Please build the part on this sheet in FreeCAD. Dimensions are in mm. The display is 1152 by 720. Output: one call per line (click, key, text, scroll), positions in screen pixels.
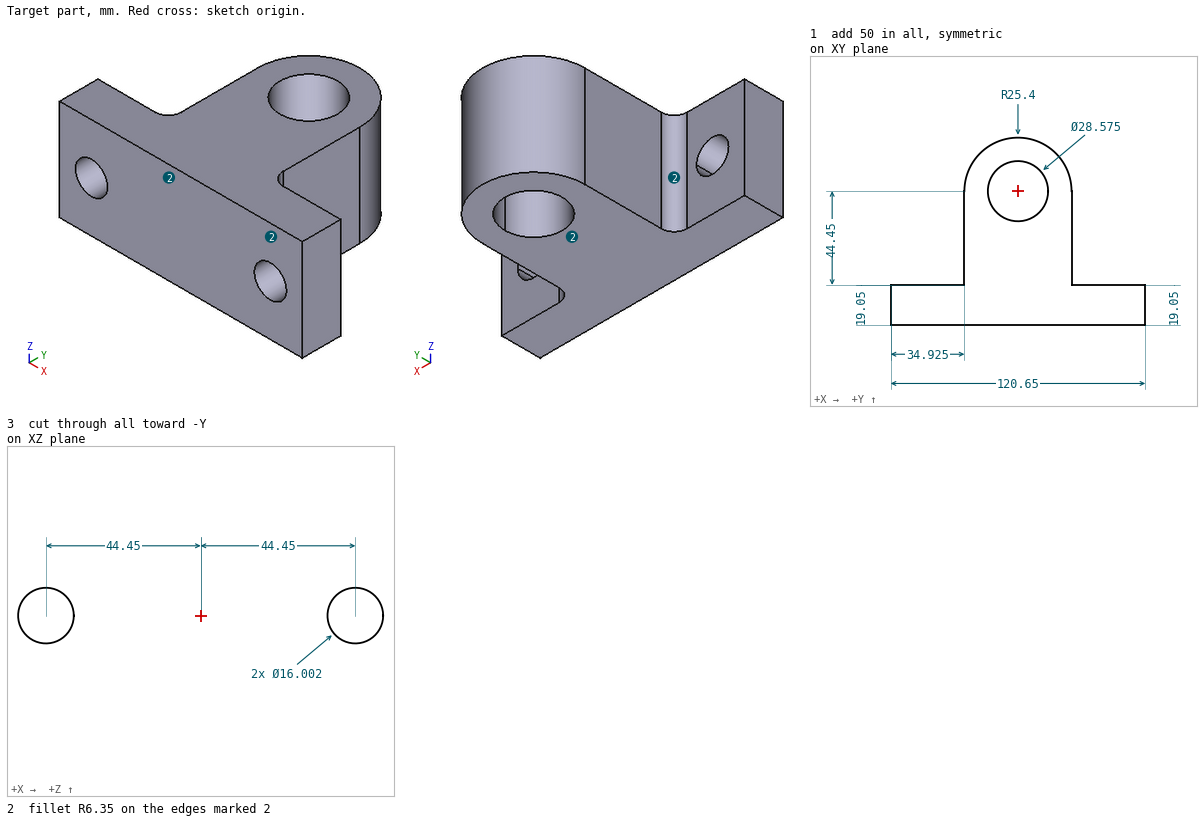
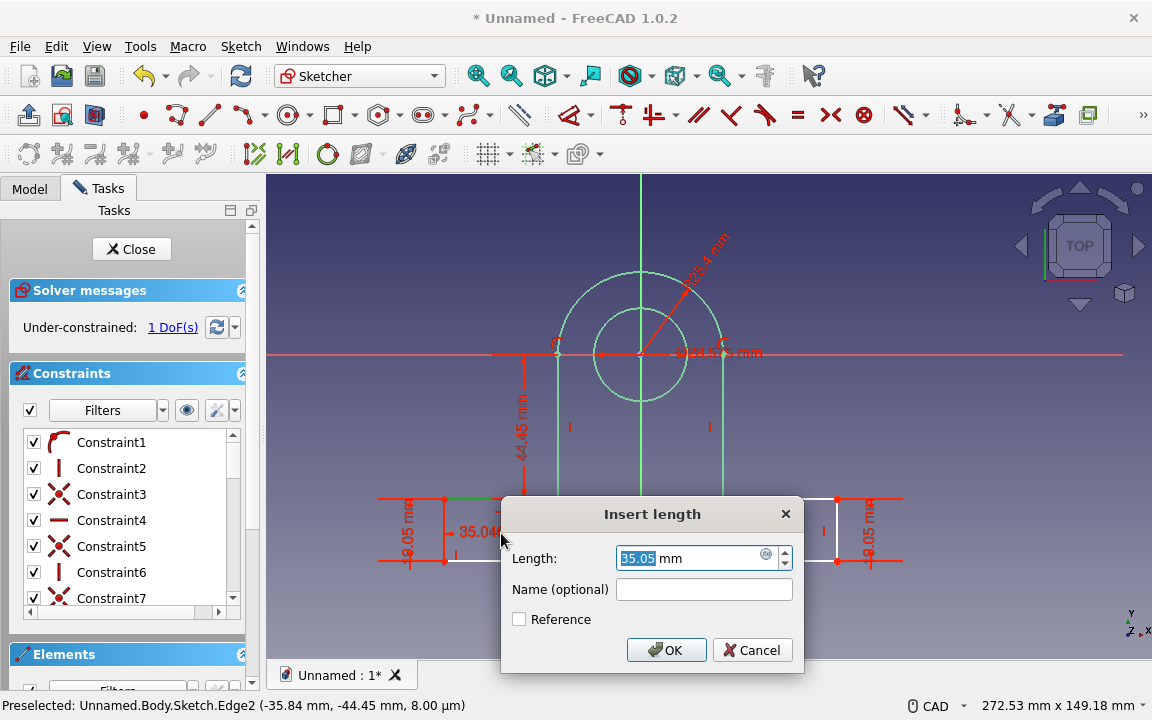
text(34.925)
key(Return)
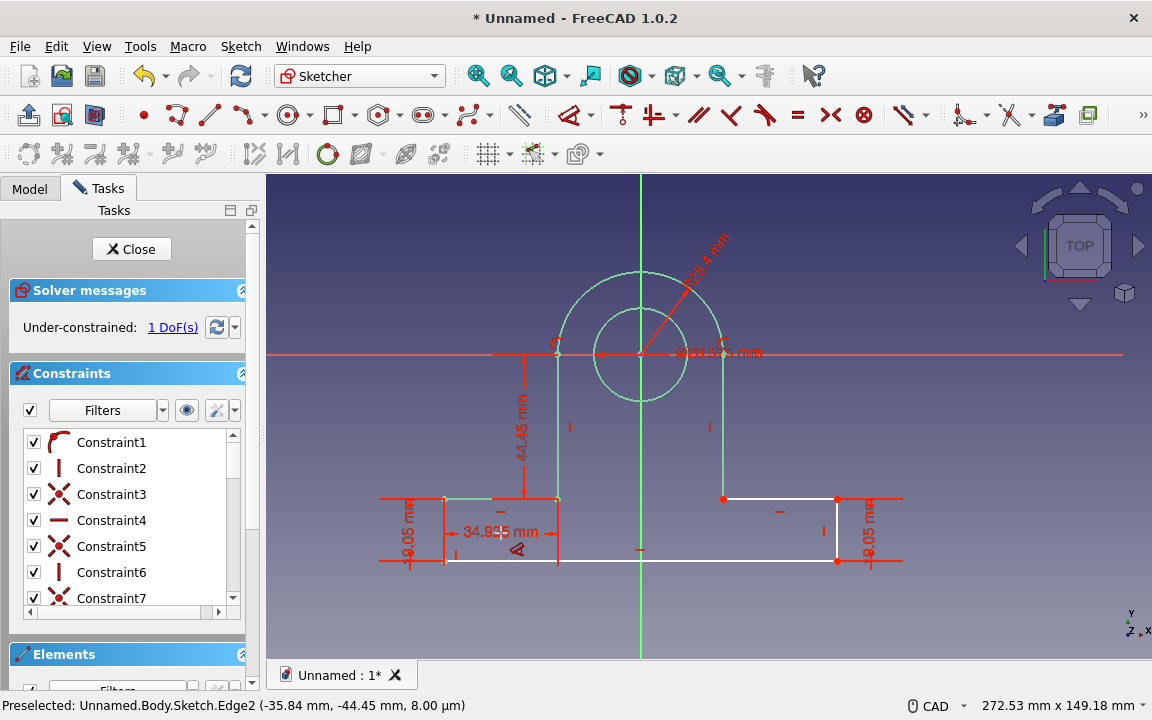
click(562, 561)
click(550, 595)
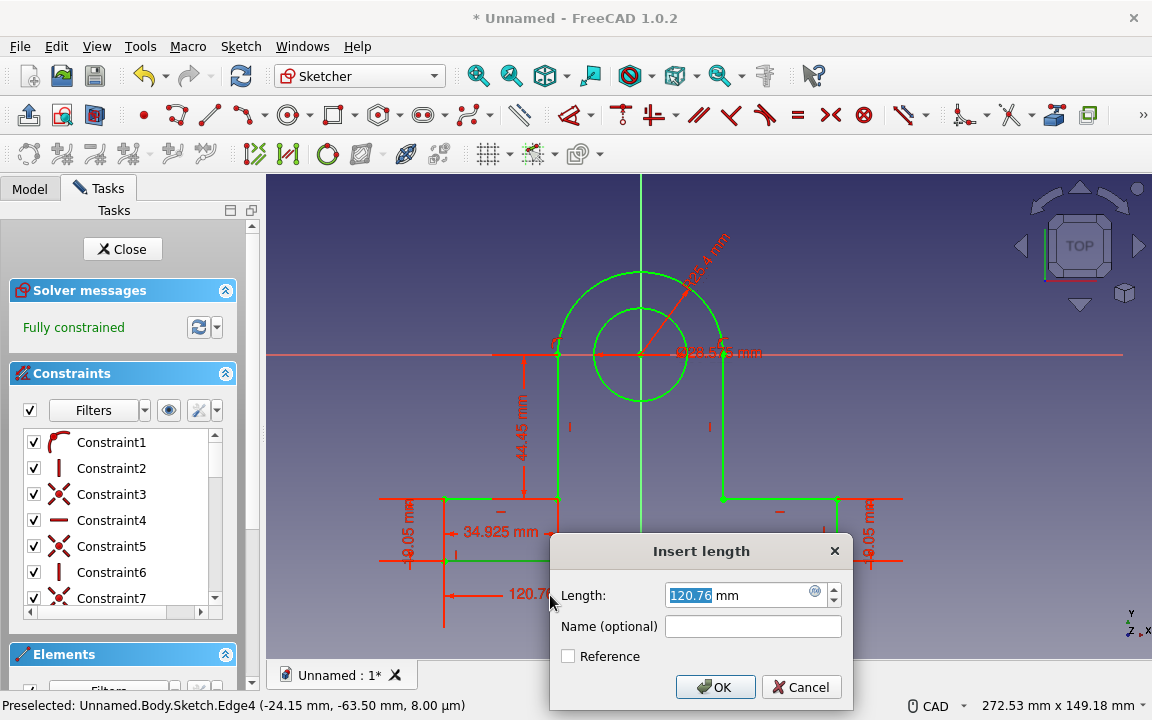
text(120.65)
key(Return)
key(Escape)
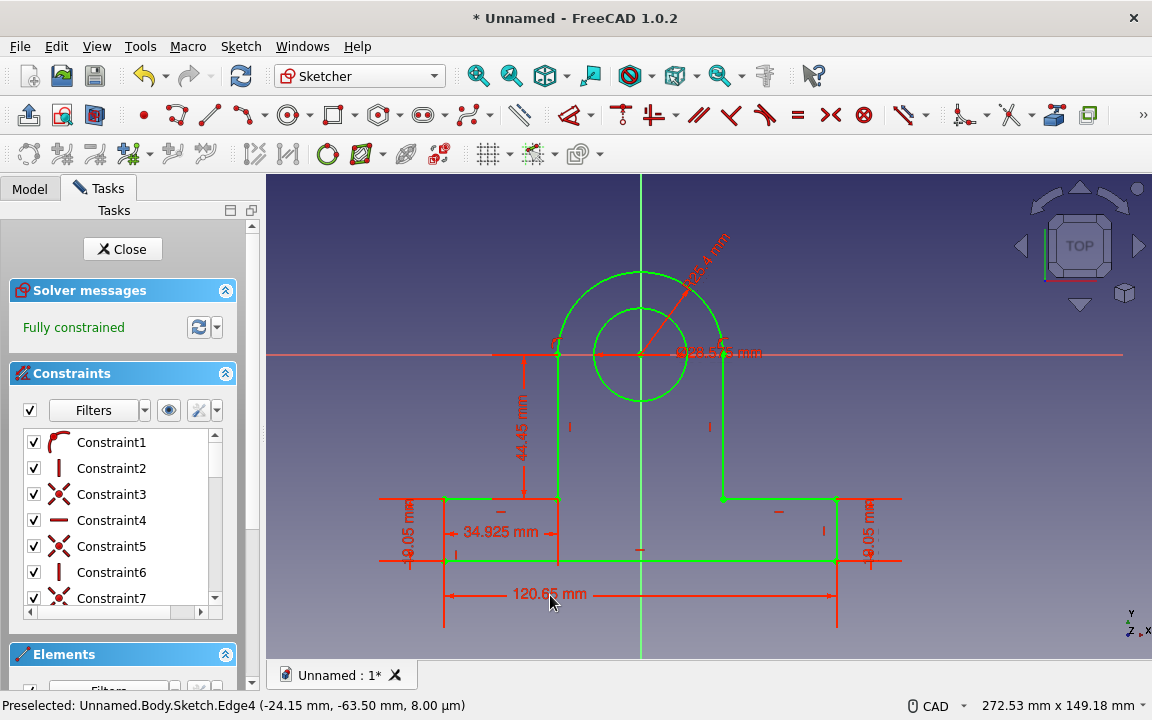
click(123, 249)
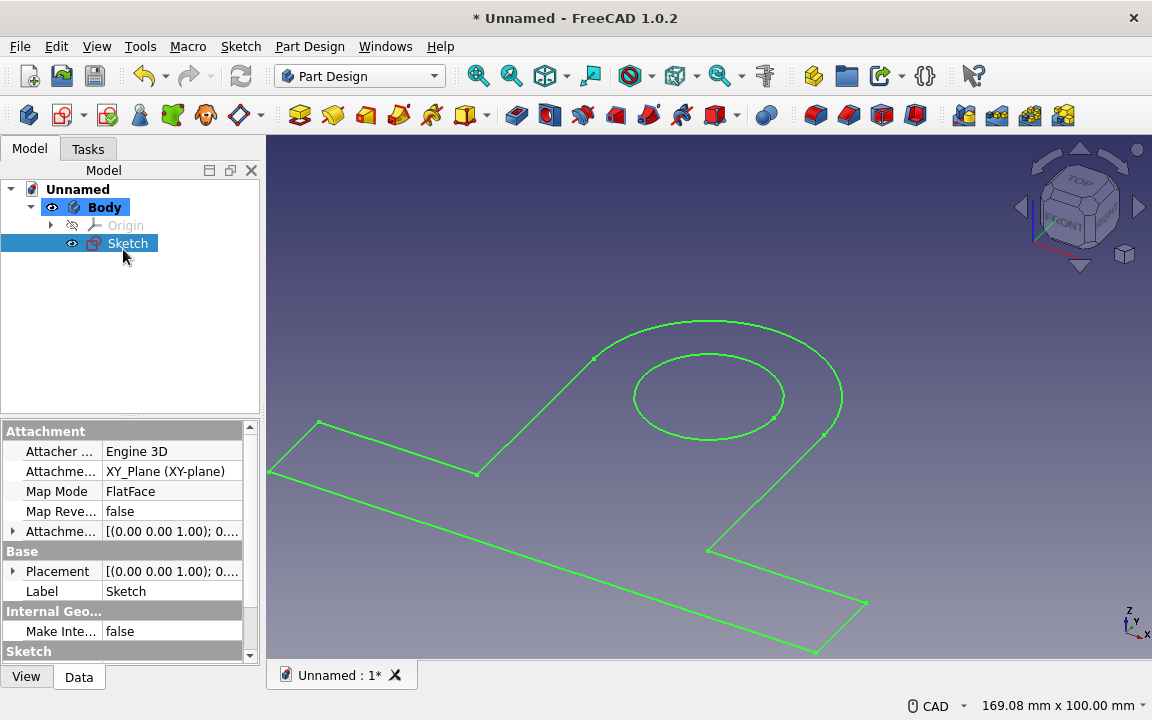
click(300, 116)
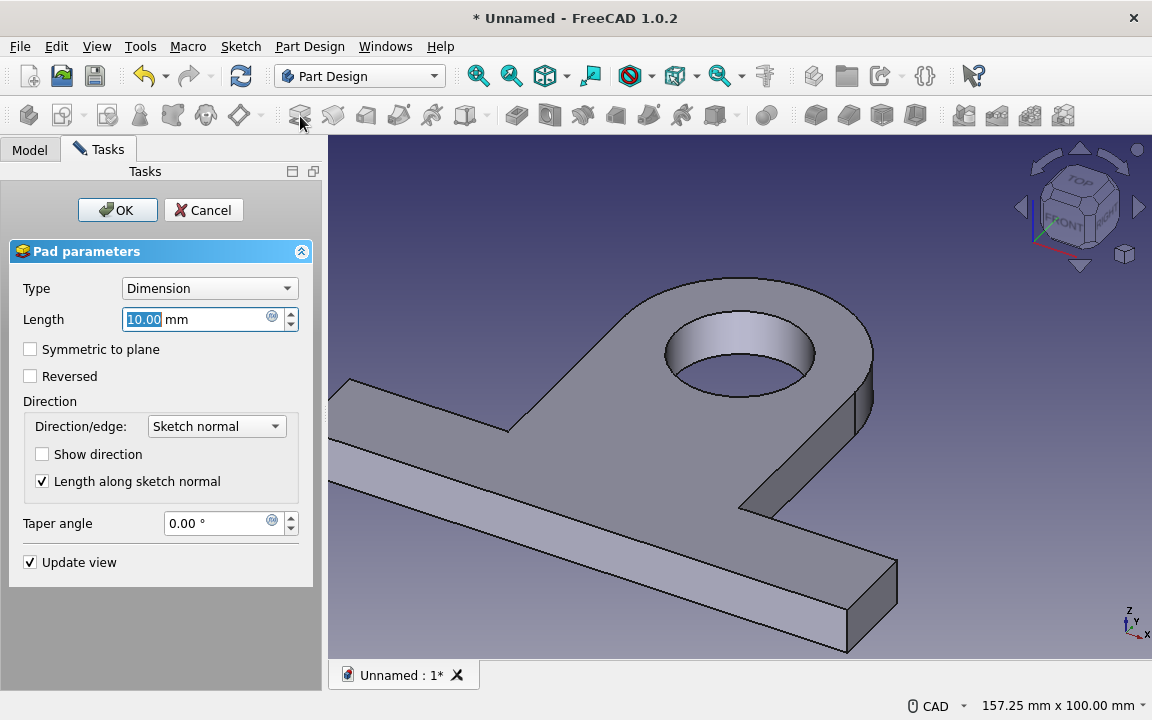
text(50)
key(Tab)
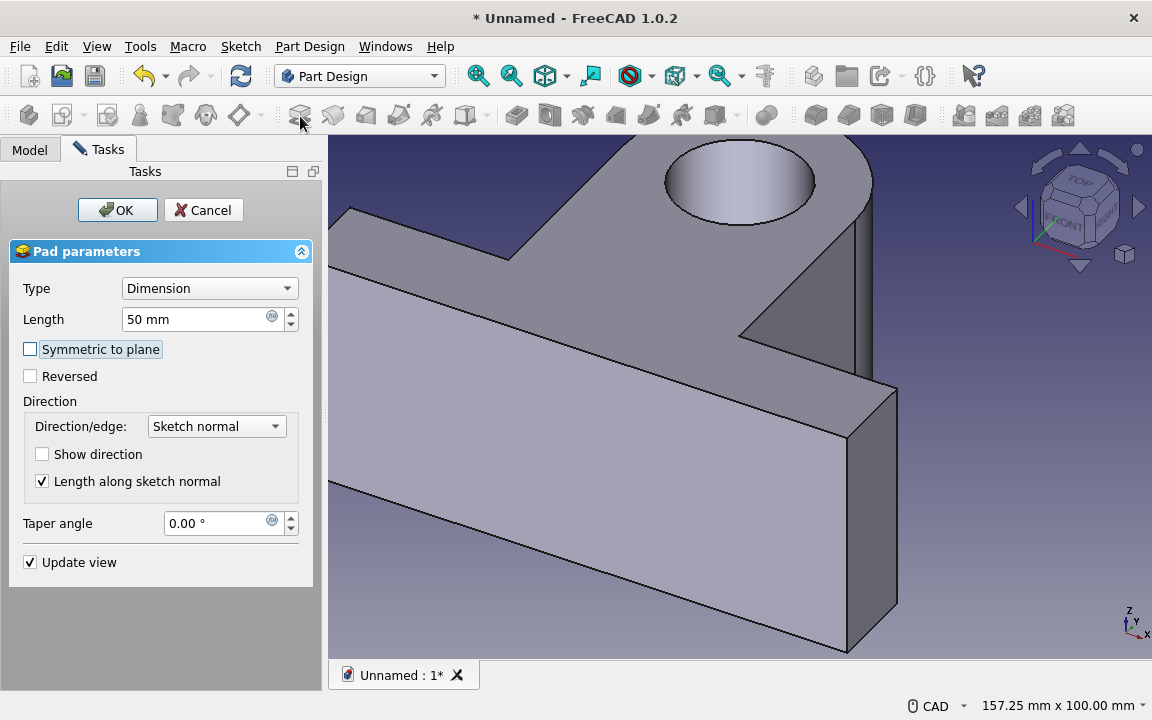
click(31, 349)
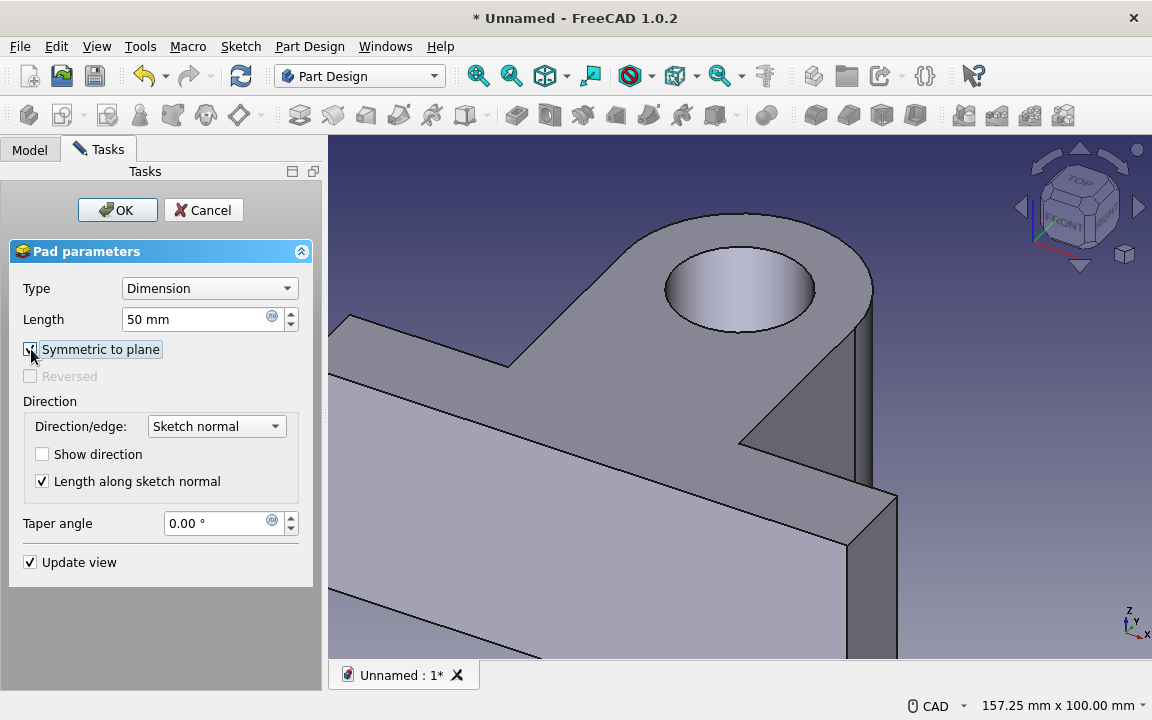
click(118, 210)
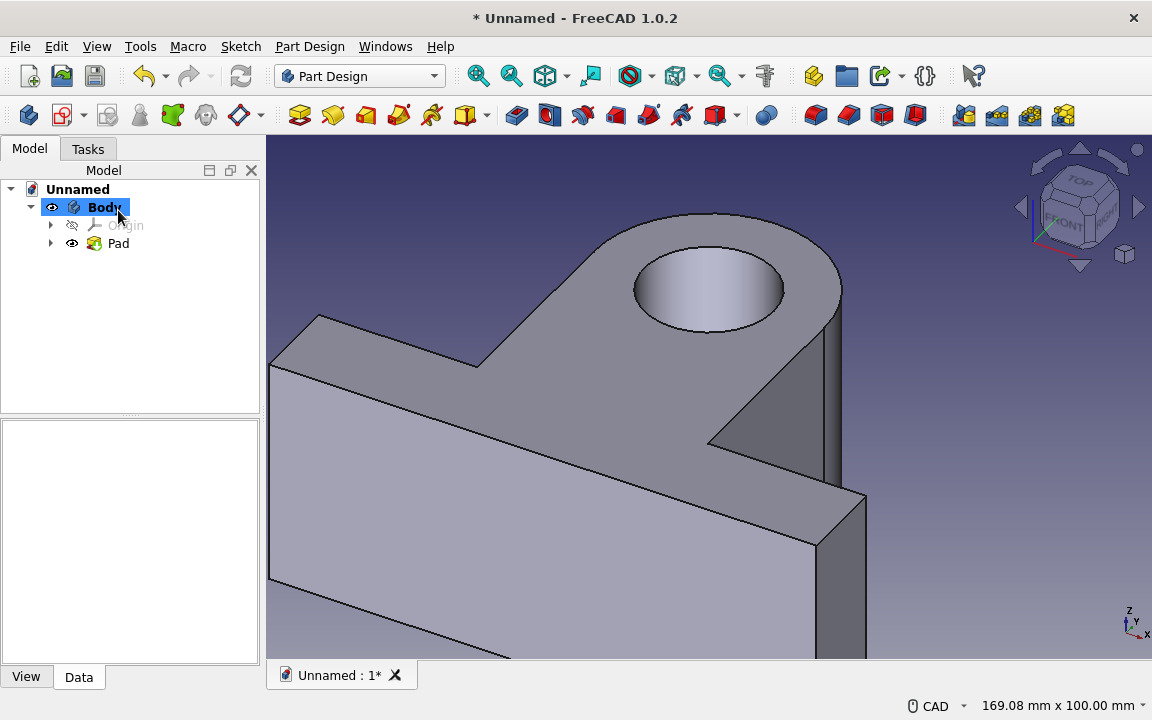
click(479, 76)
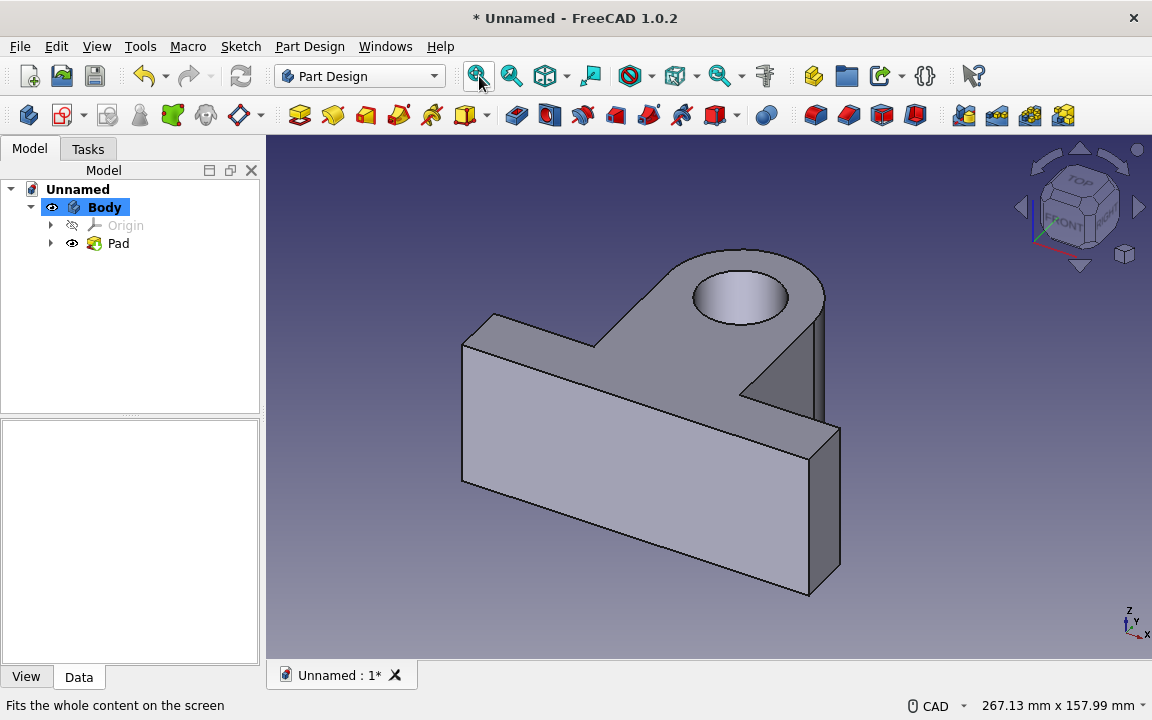
key(0)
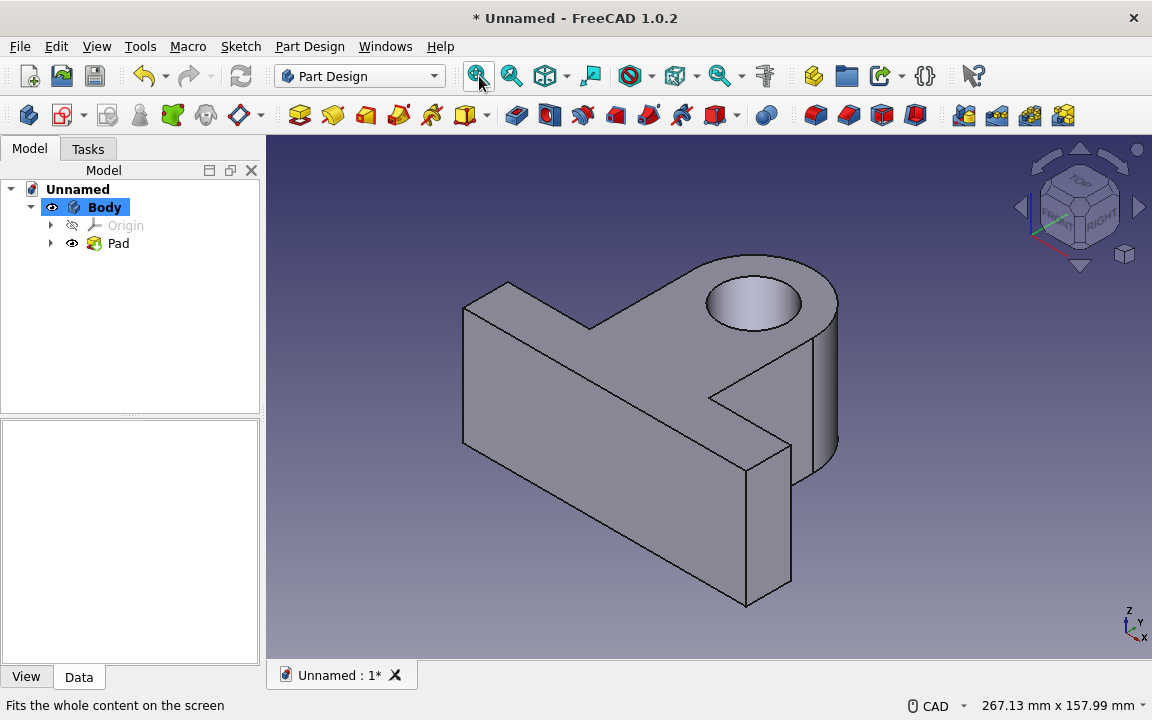
key(2)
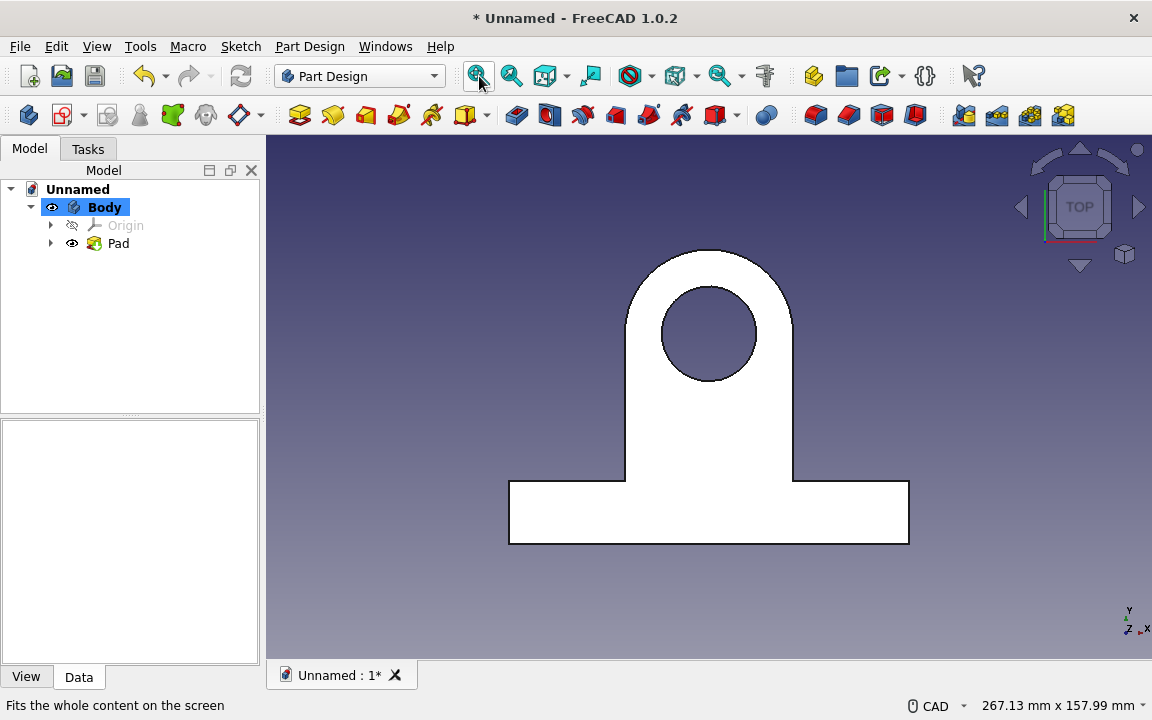
key(1)